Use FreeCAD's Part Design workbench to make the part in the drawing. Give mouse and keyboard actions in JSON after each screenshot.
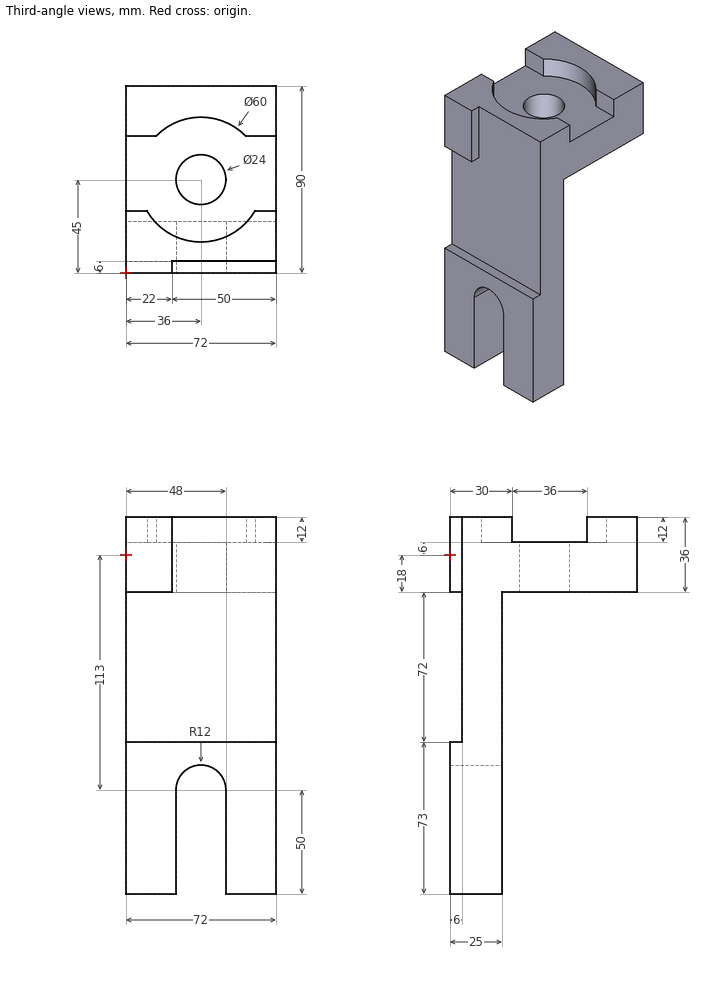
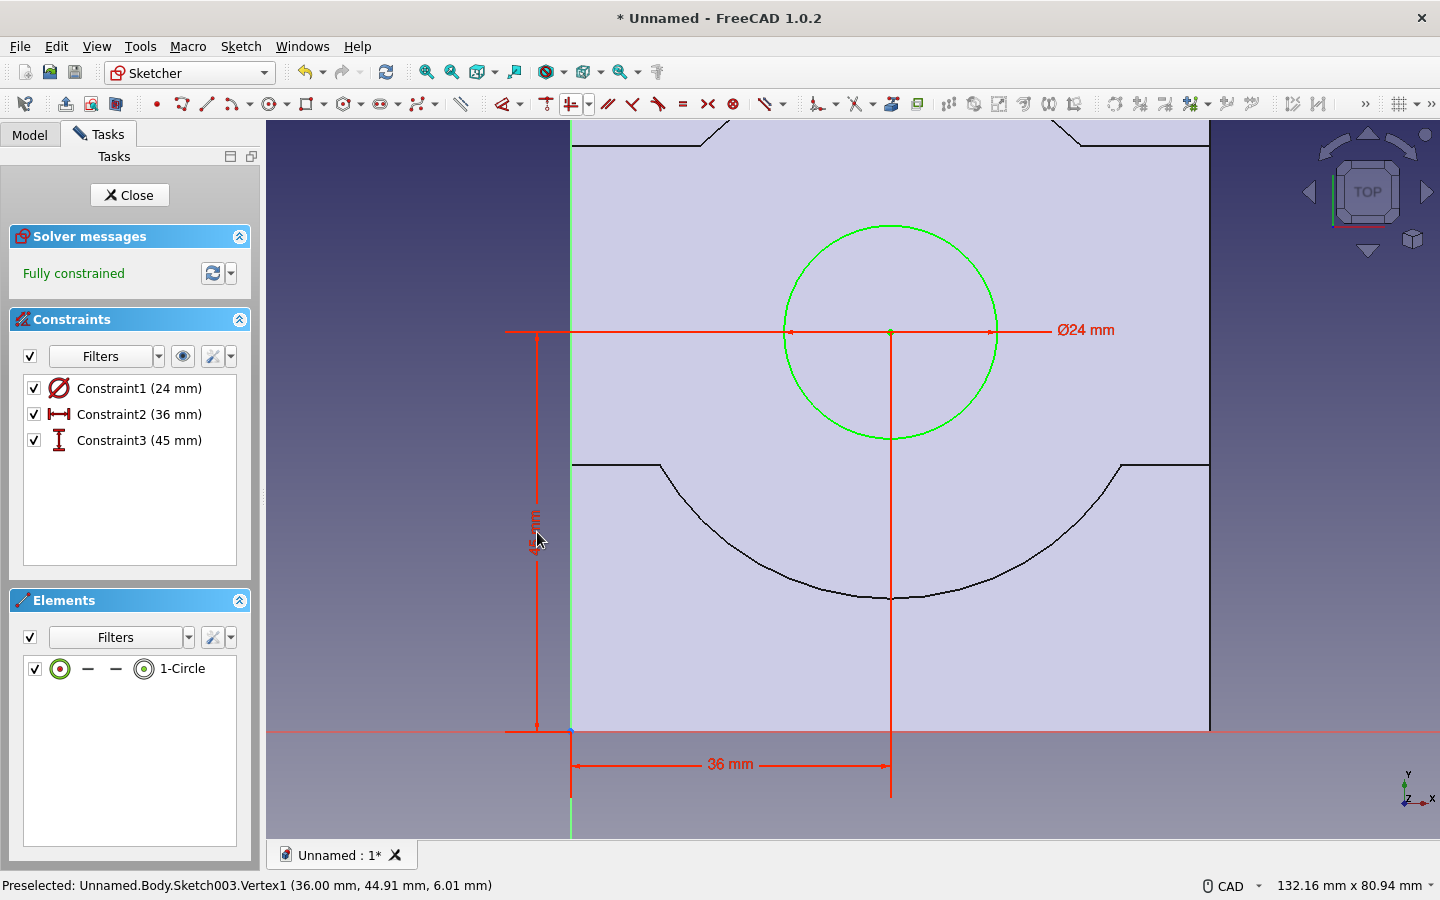
{"action": "left_click", "coordinate": [130, 195]}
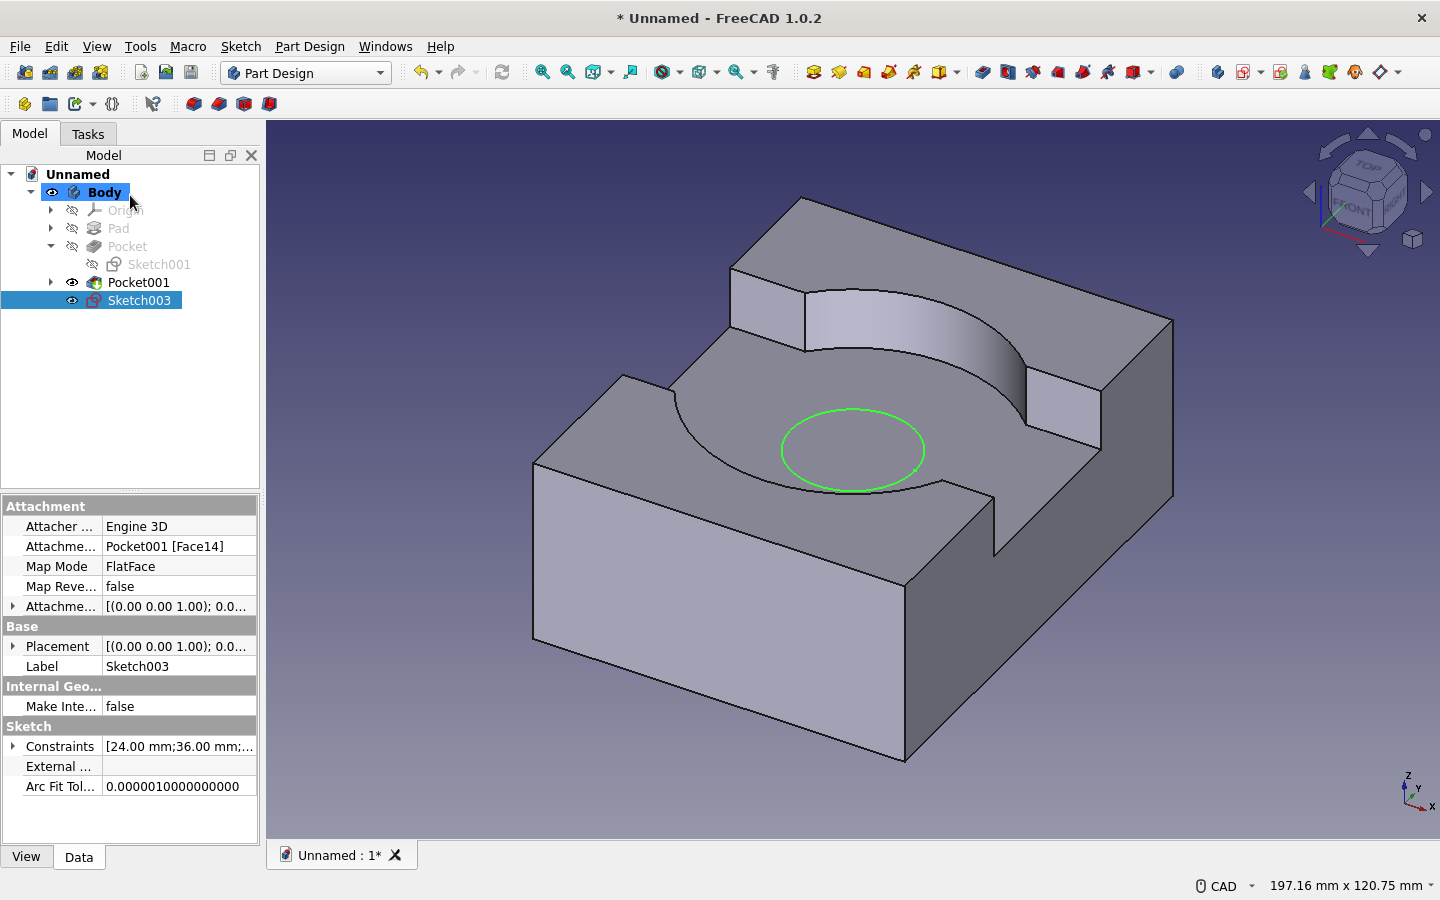
{"action": "left_click", "coordinate": [983, 72]}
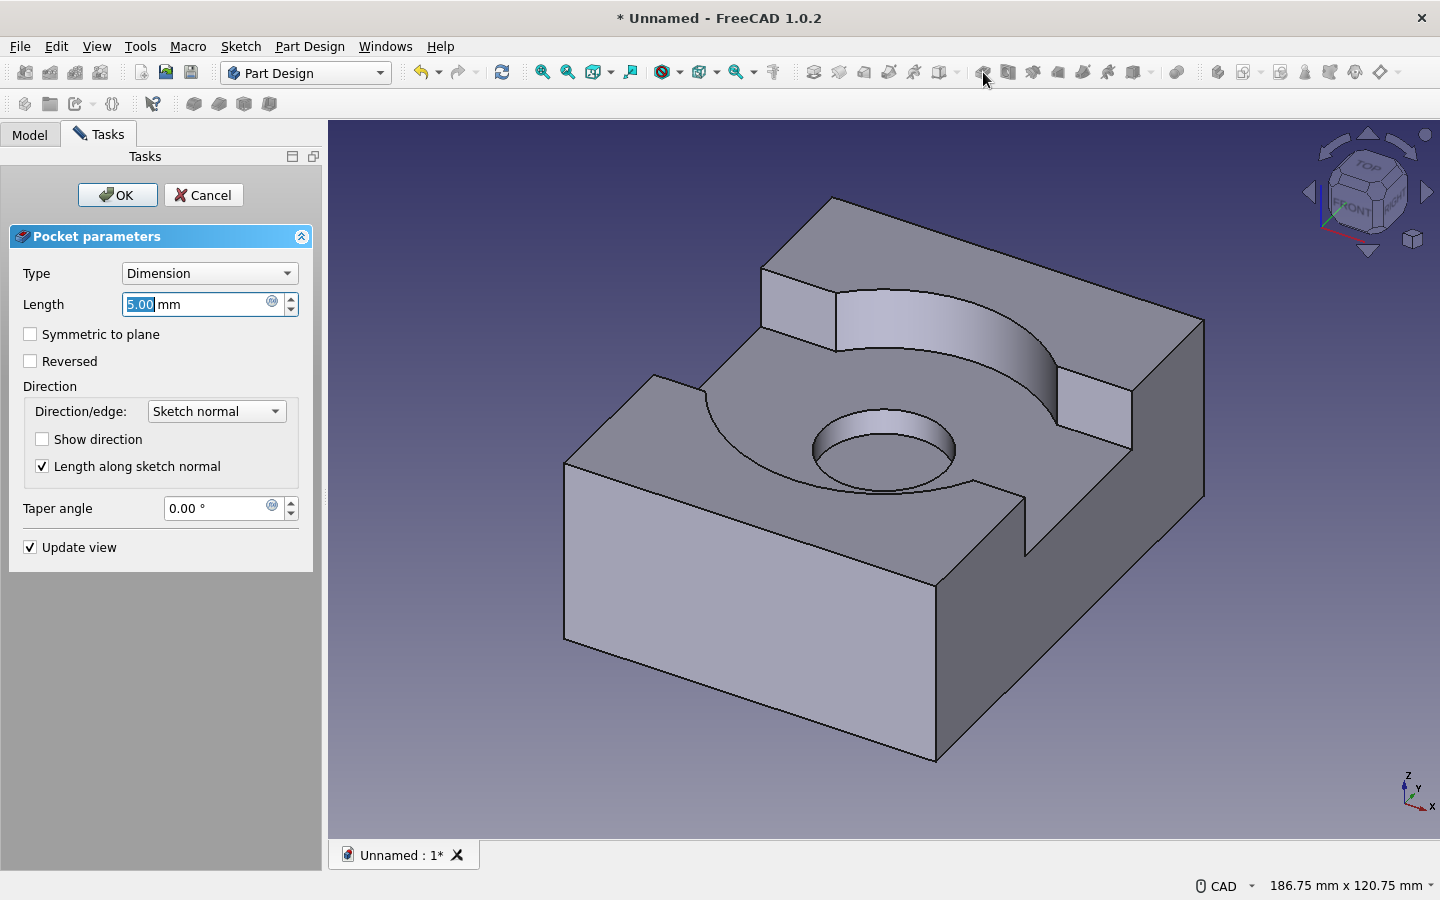
{"action": "left_click", "coordinate": [210, 274]}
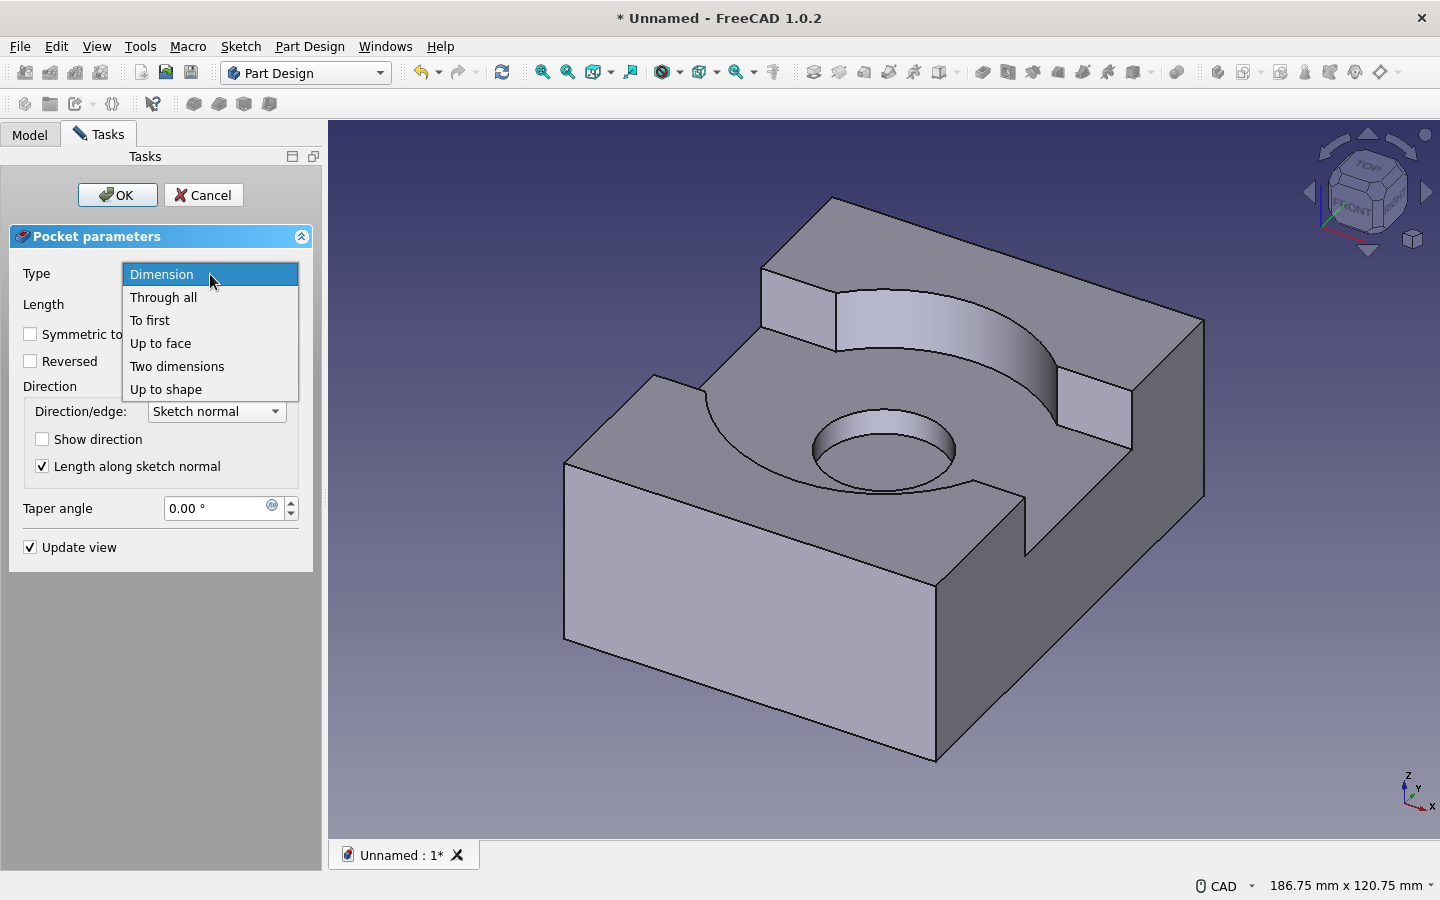
{"action": "left_click", "coordinate": [208, 298]}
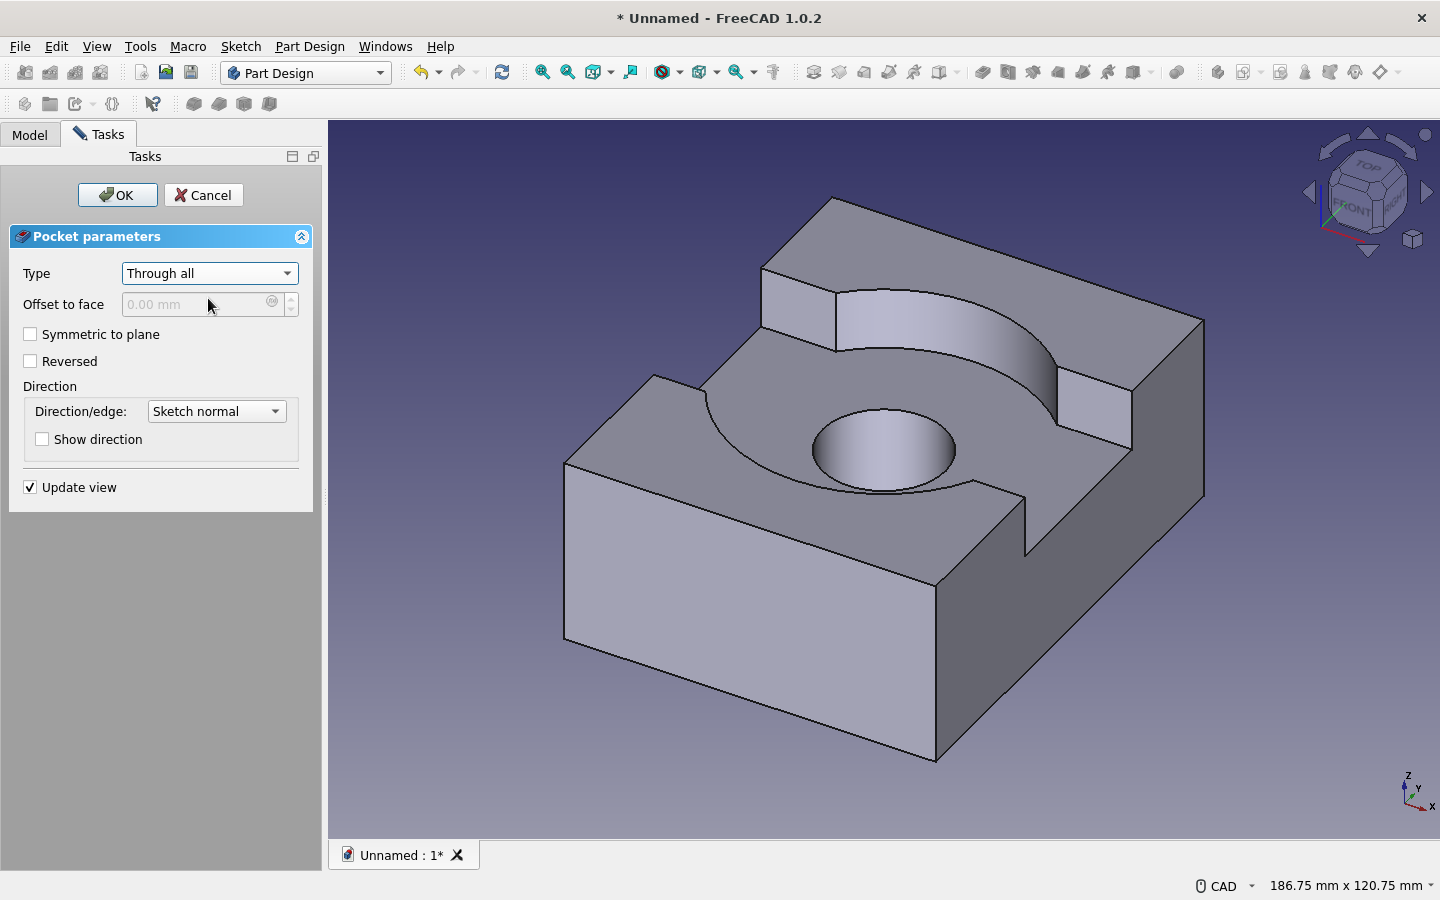
{"action": "left_click", "coordinate": [118, 195]}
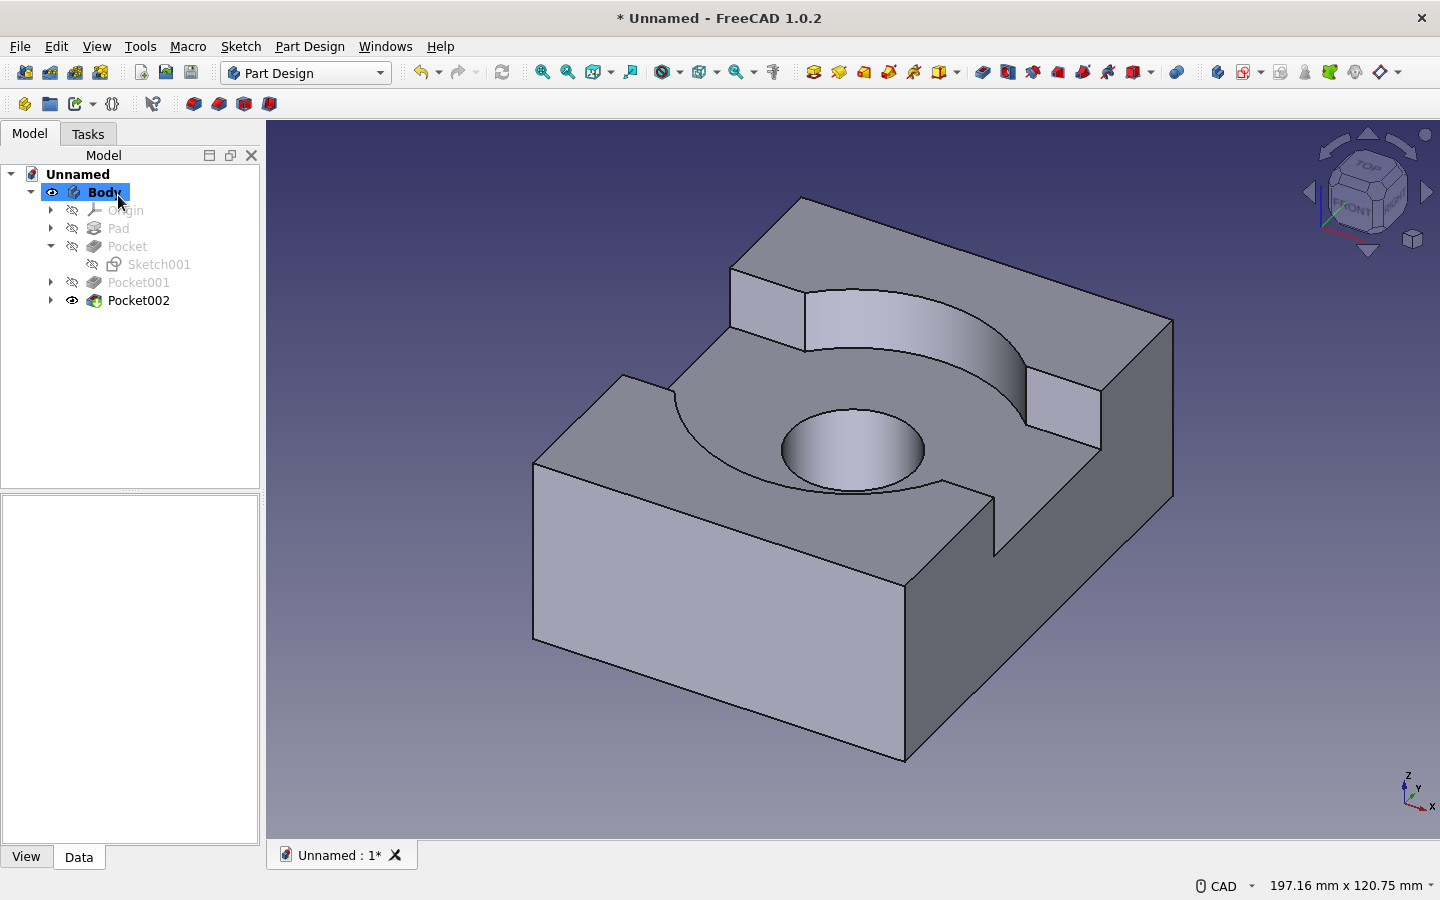
{"action": "left_click", "coordinate": [645, 457]}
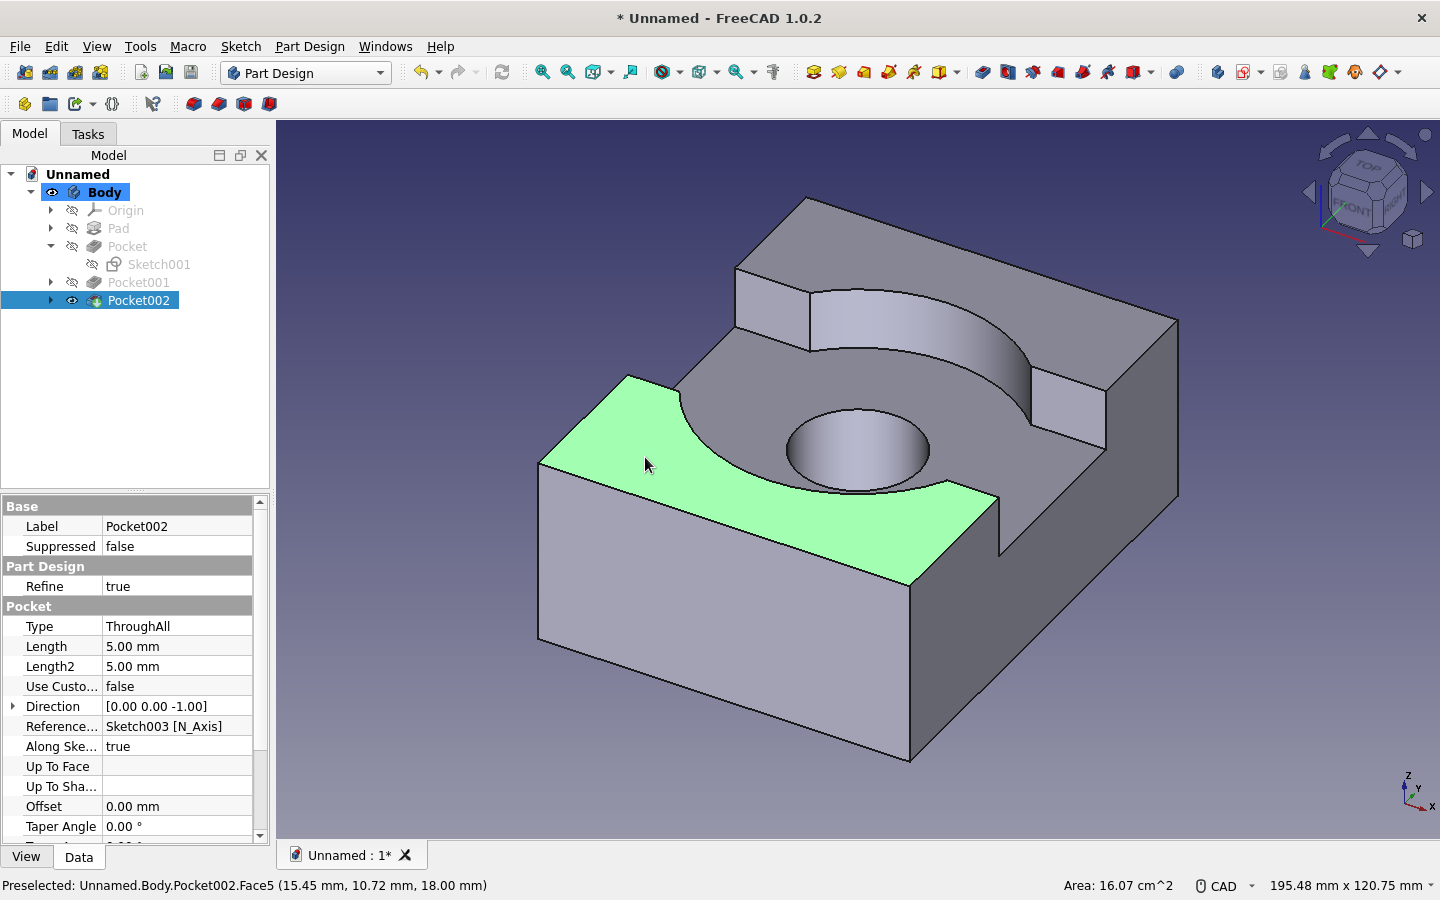
{"action": "left_click", "coordinate": [1242, 72]}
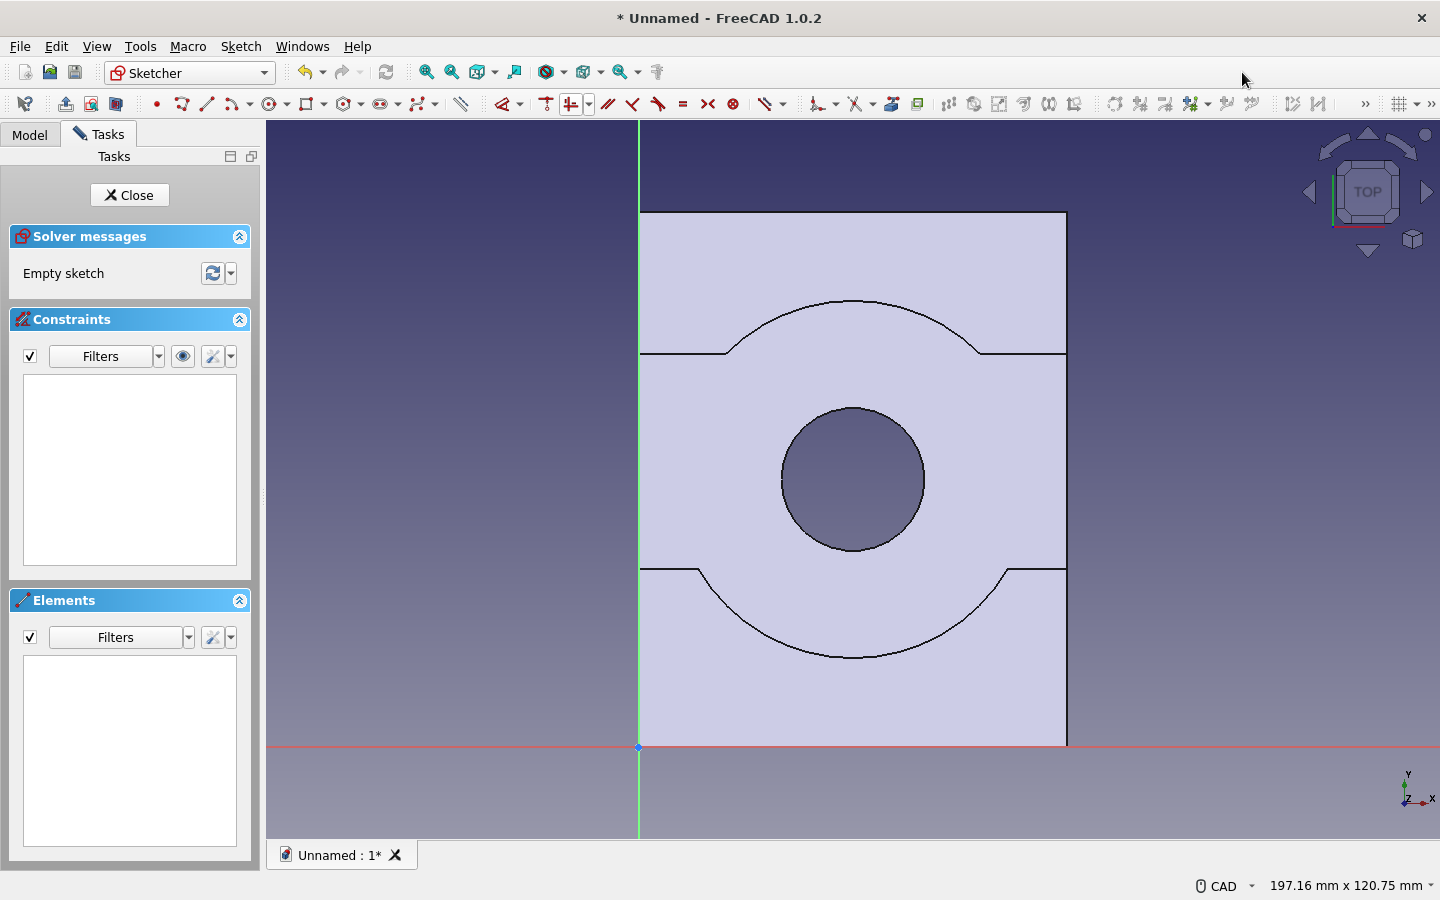
{"action": "scroll", "coordinate": [992, 811], "scroll_direction": "up", "scroll_amount": 2}